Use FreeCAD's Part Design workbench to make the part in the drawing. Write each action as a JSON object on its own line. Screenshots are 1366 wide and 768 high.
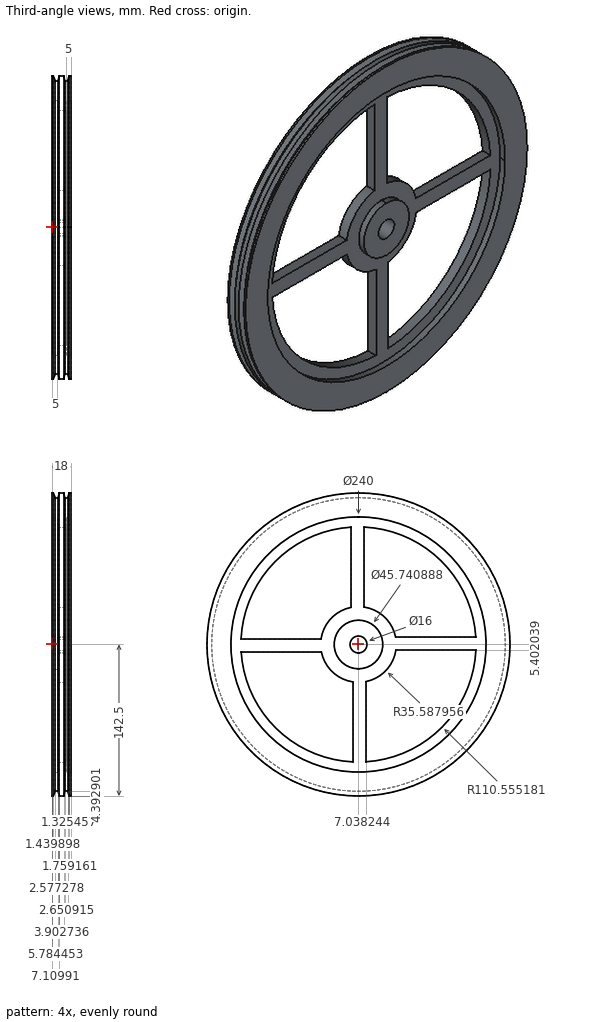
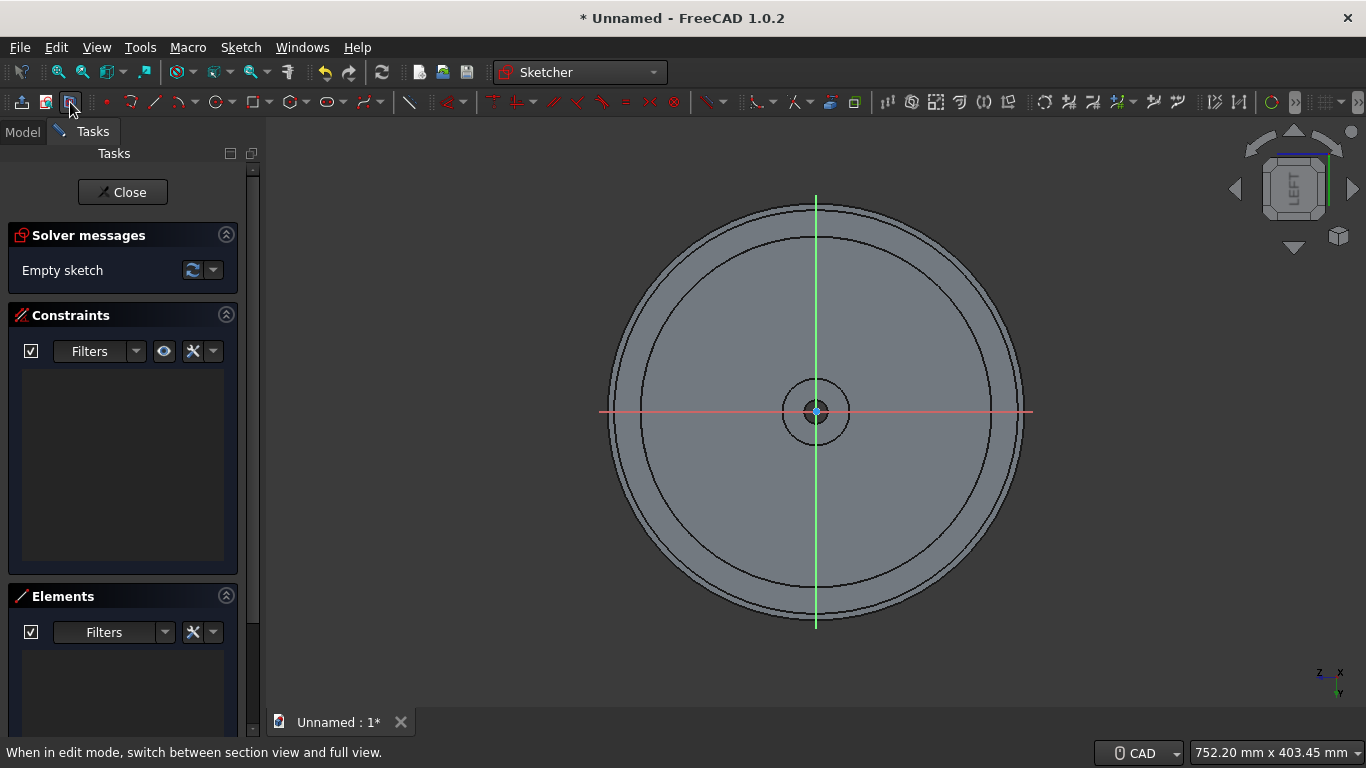
{"action": "scroll", "coordinate": [1018, 559], "scroll_direction": "up", "scroll_amount": 4}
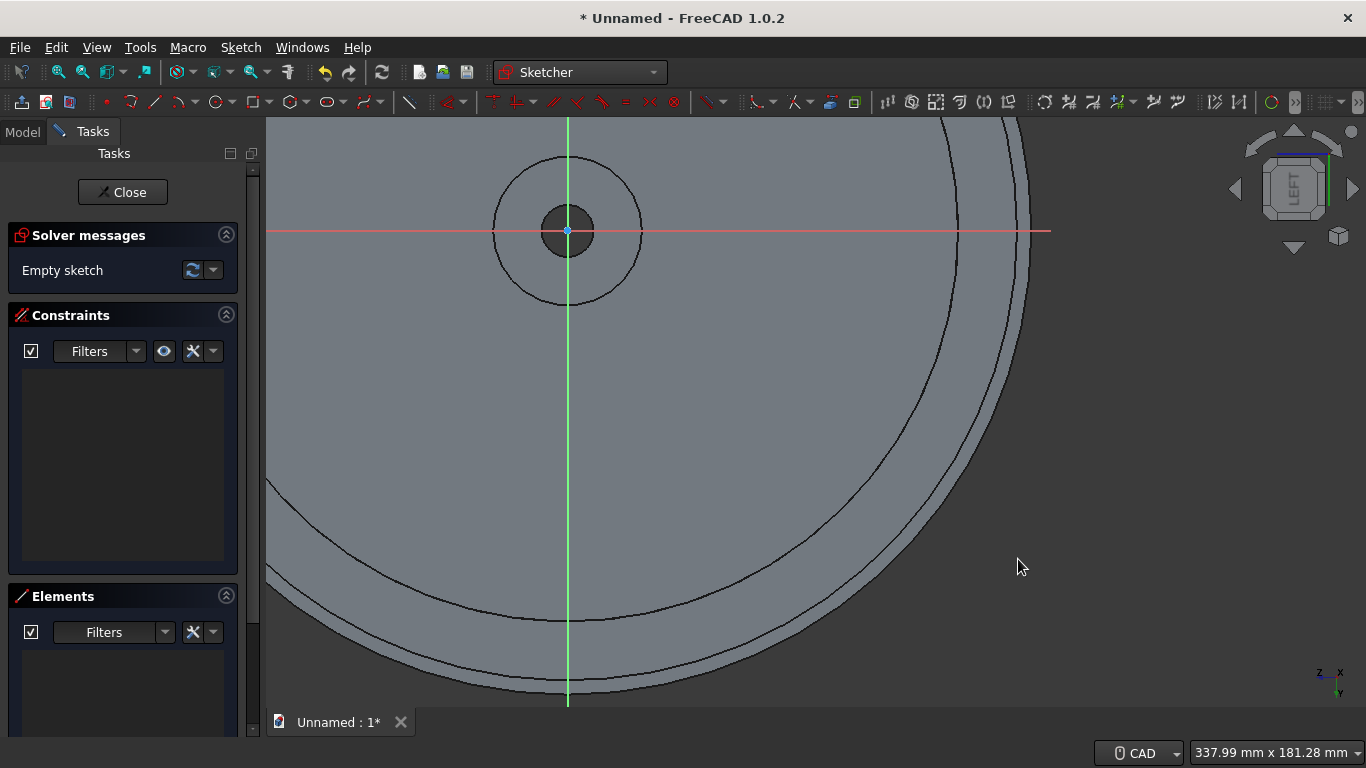
{"action": "key", "text": "g l"}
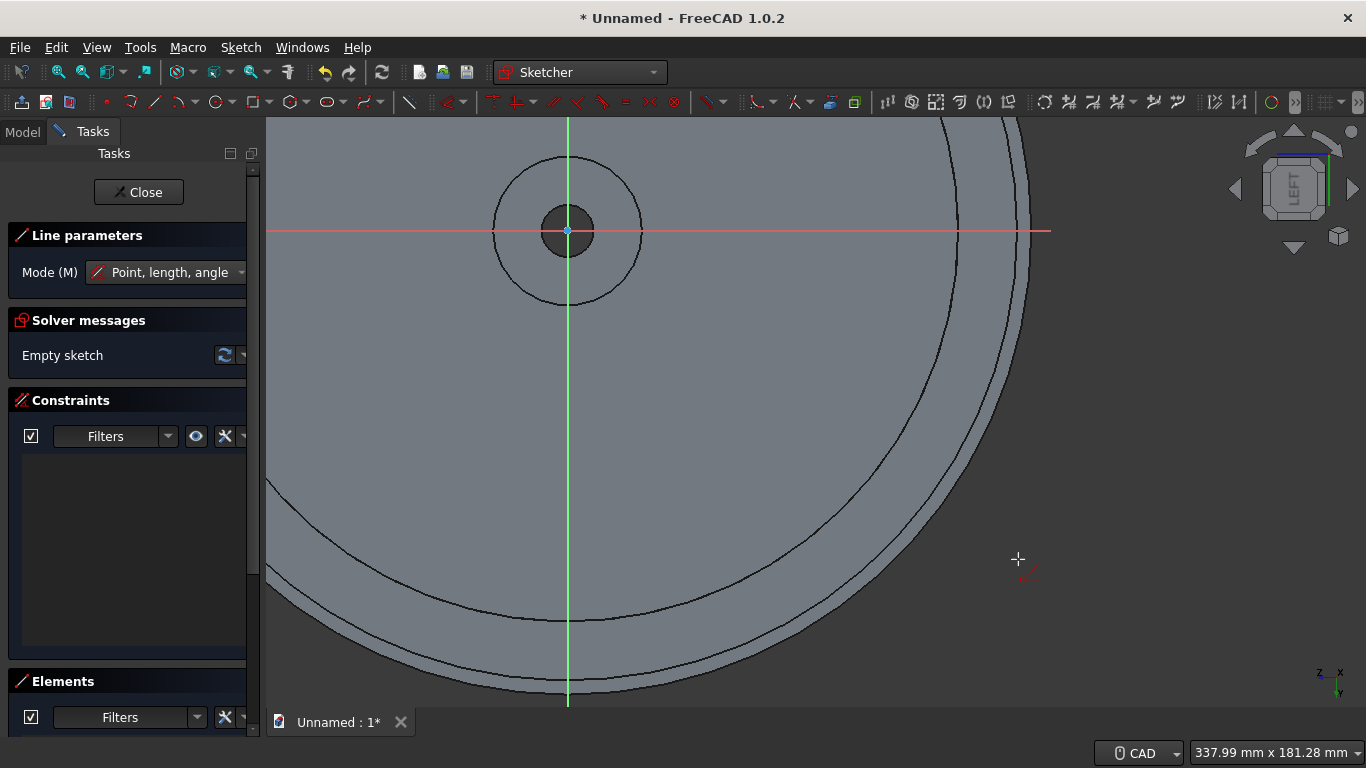
{"action": "left_click", "coordinate": [585, 345]}
{"action": "left_click", "coordinate": [585, 590]}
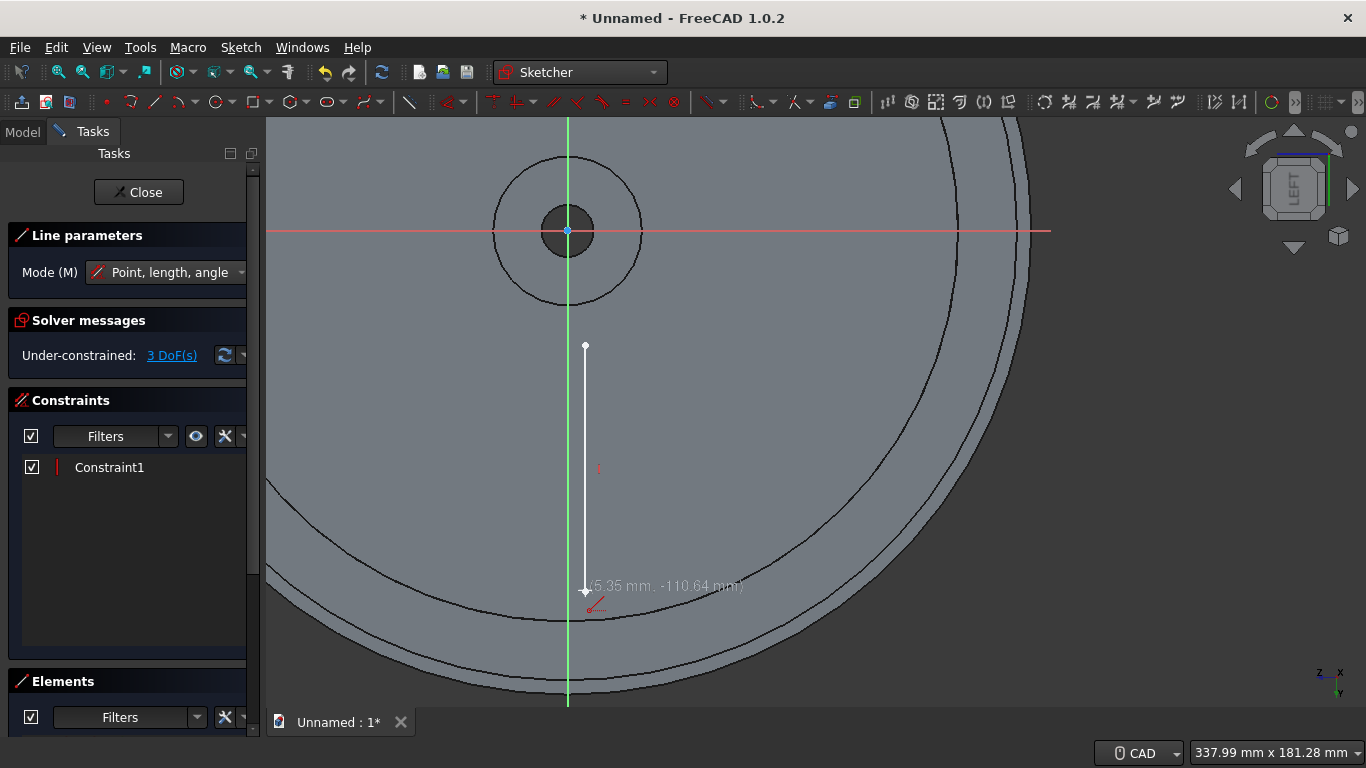
{"action": "left_click", "coordinate": [927, 254]}
{"action": "left_click", "coordinate": [681, 254]}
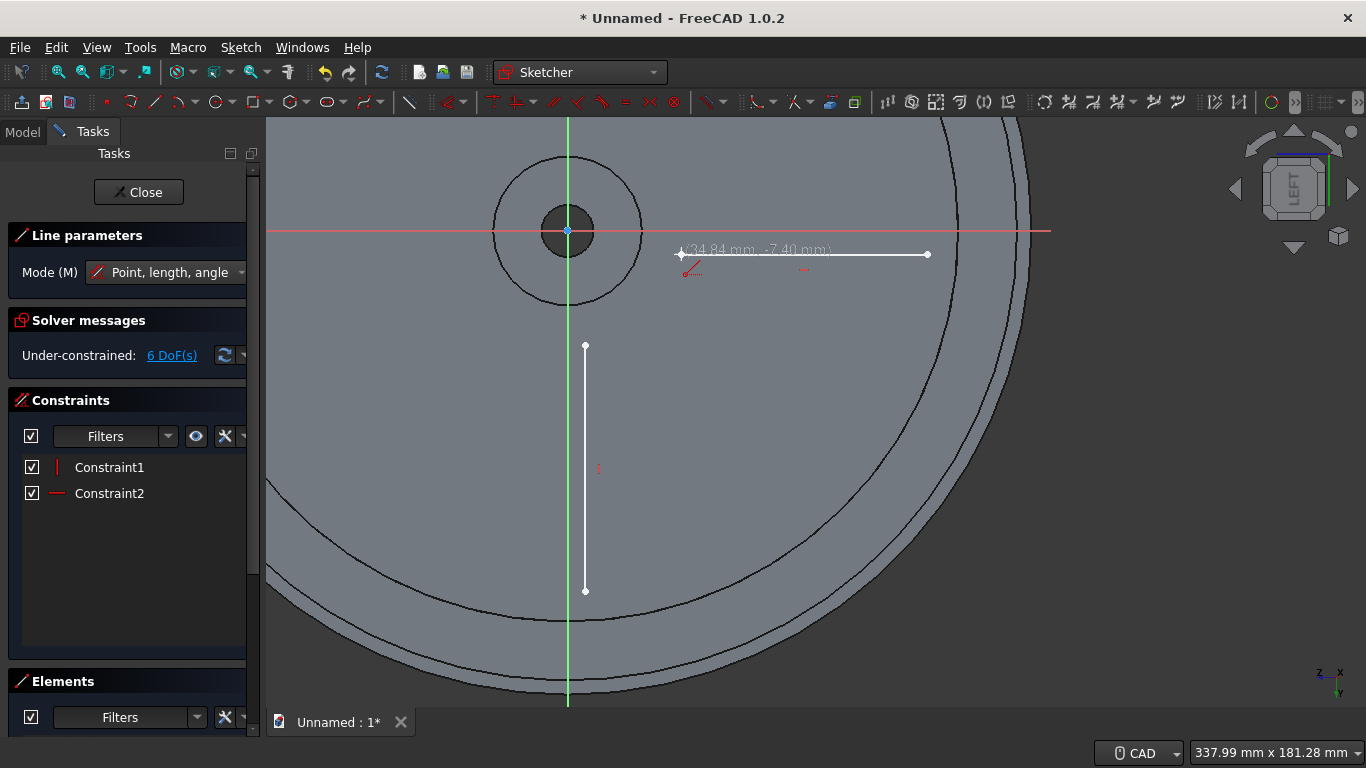
{"action": "key", "text": "g 3 a"}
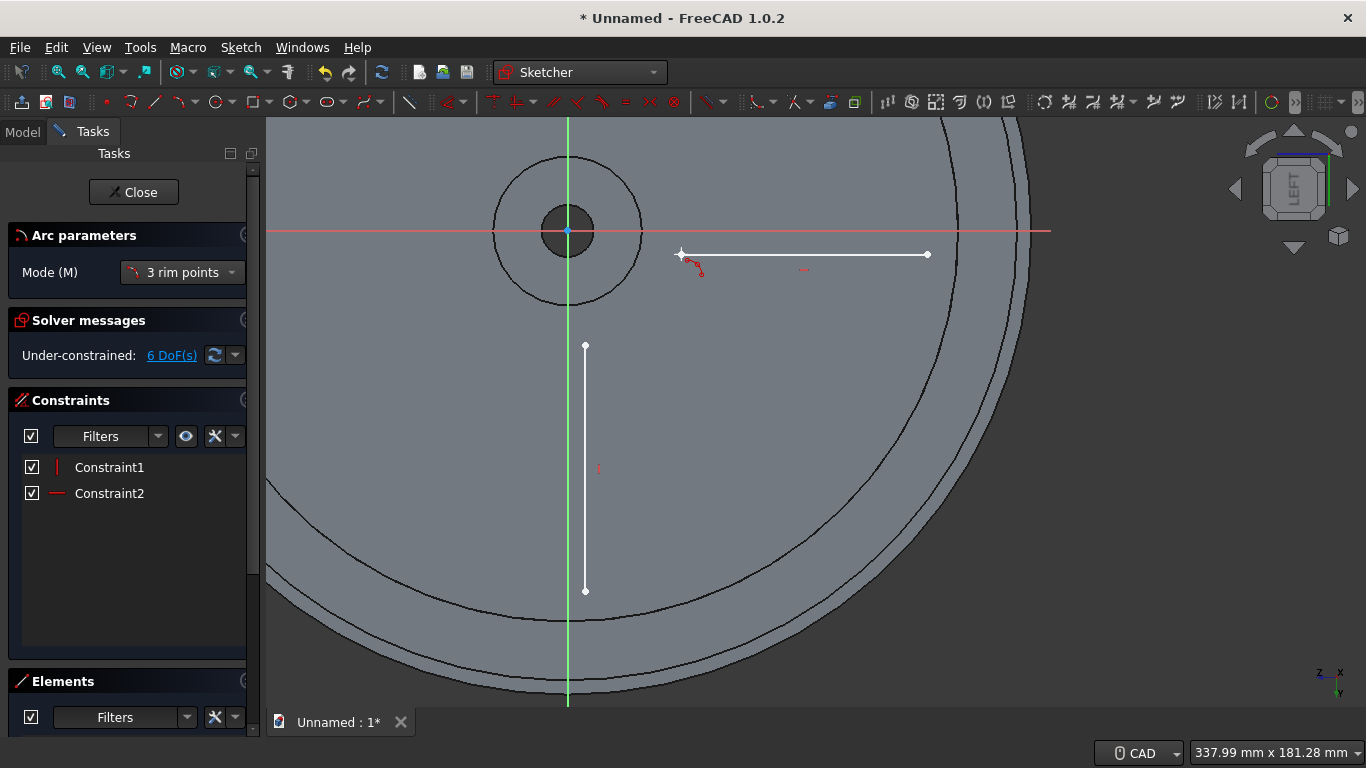
{"action": "left_click", "coordinate": [585, 591]}
{"action": "left_click", "coordinate": [927, 255]}
{"action": "left_click", "coordinate": [820, 487]}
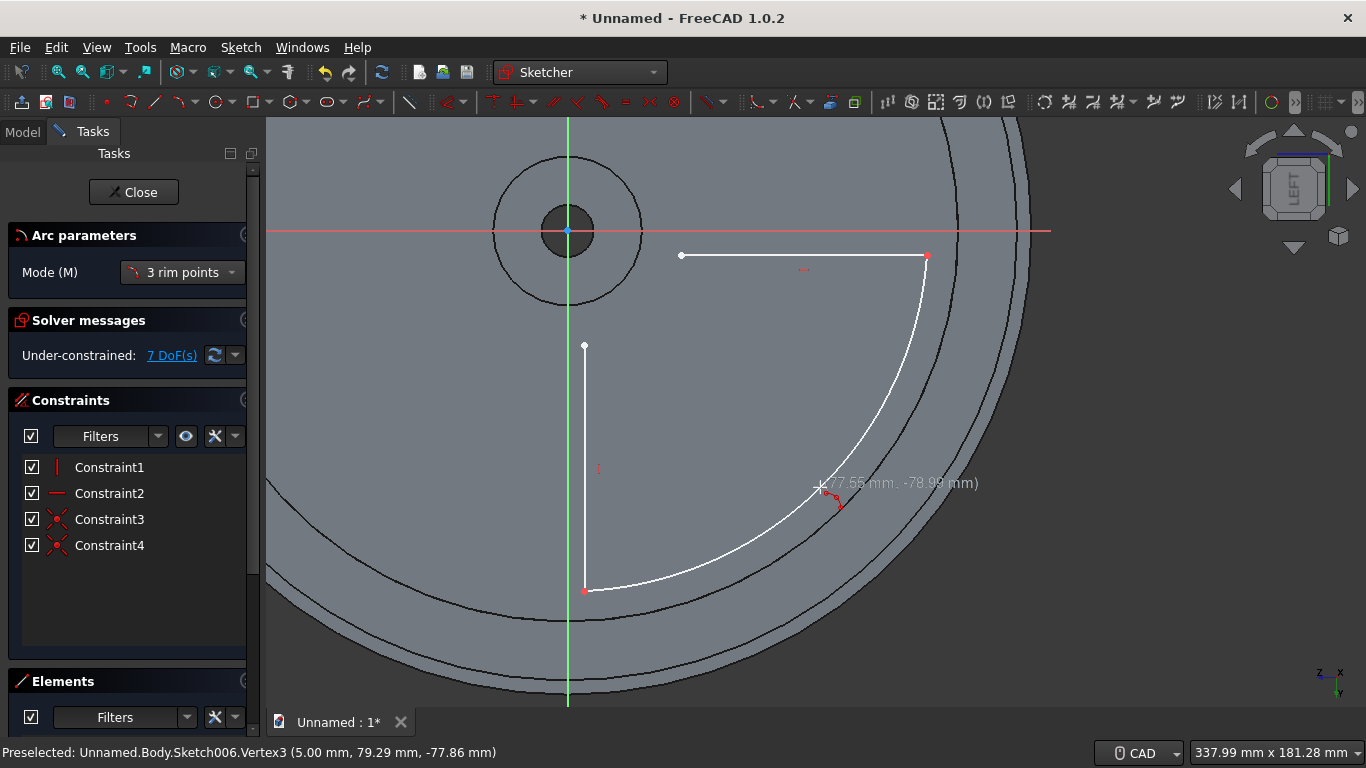
{"action": "left_click", "coordinate": [681, 255]}
{"action": "left_click", "coordinate": [585, 346]}
{"action": "left_click", "coordinate": [648, 315]}
{"action": "key", "text": "Escape"}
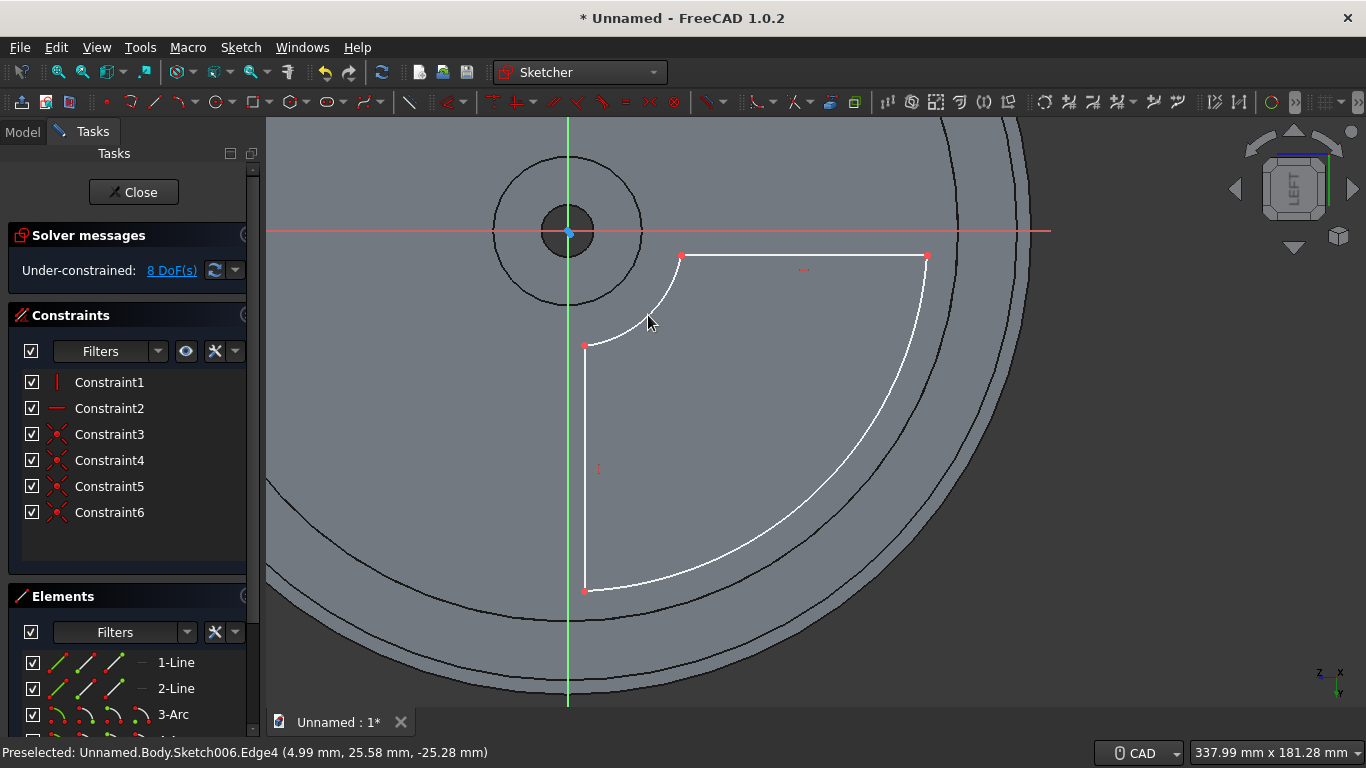
{"action": "left_click", "coordinate": [736, 550]}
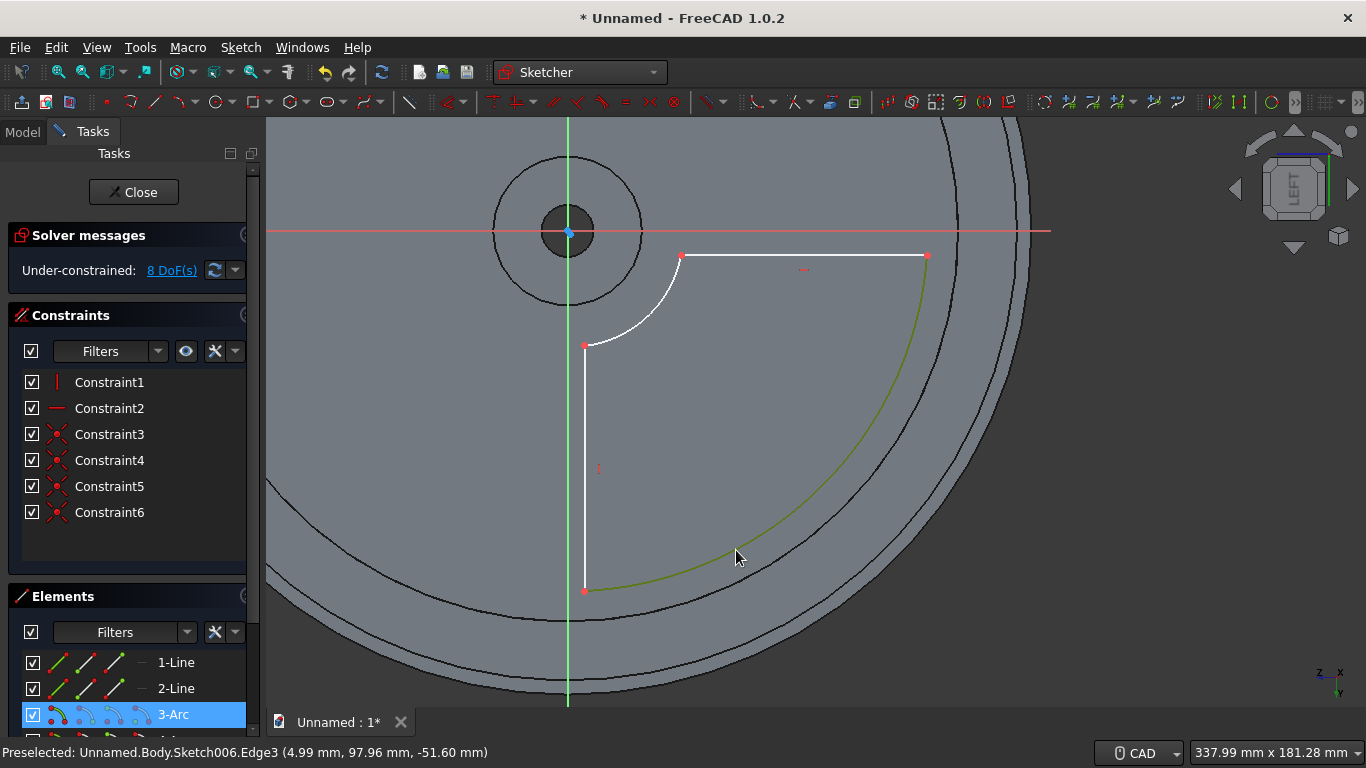
{"action": "left_click", "coordinate": [625, 333]}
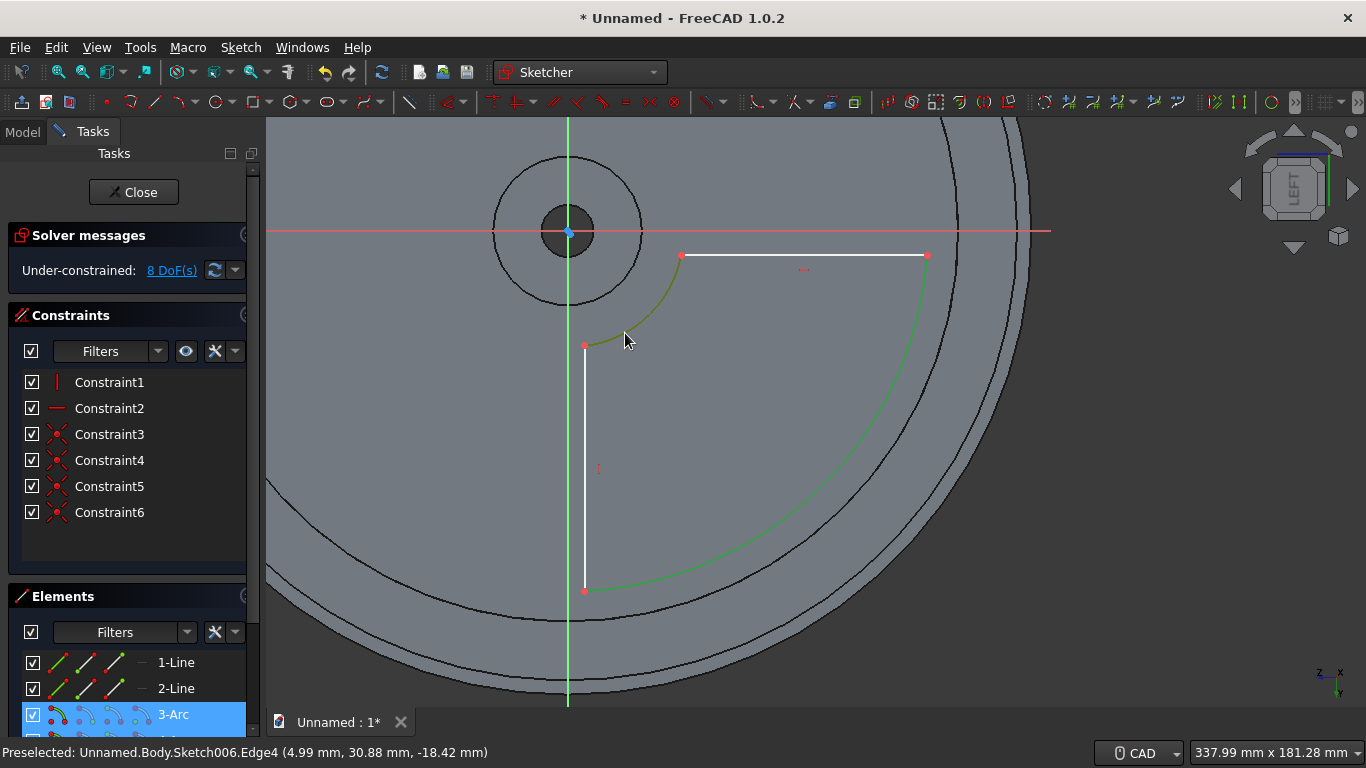
{"action": "left_click", "coordinate": [494, 102]}